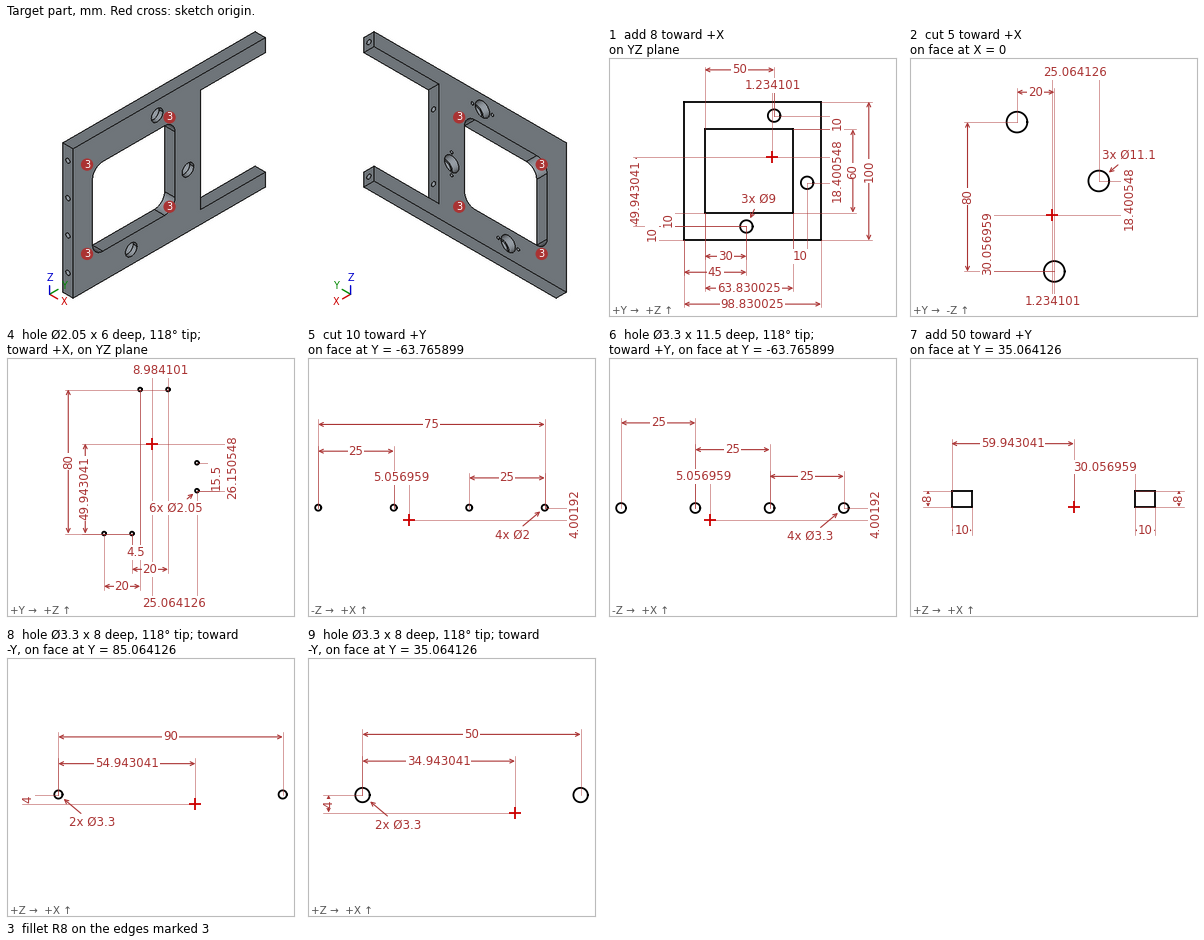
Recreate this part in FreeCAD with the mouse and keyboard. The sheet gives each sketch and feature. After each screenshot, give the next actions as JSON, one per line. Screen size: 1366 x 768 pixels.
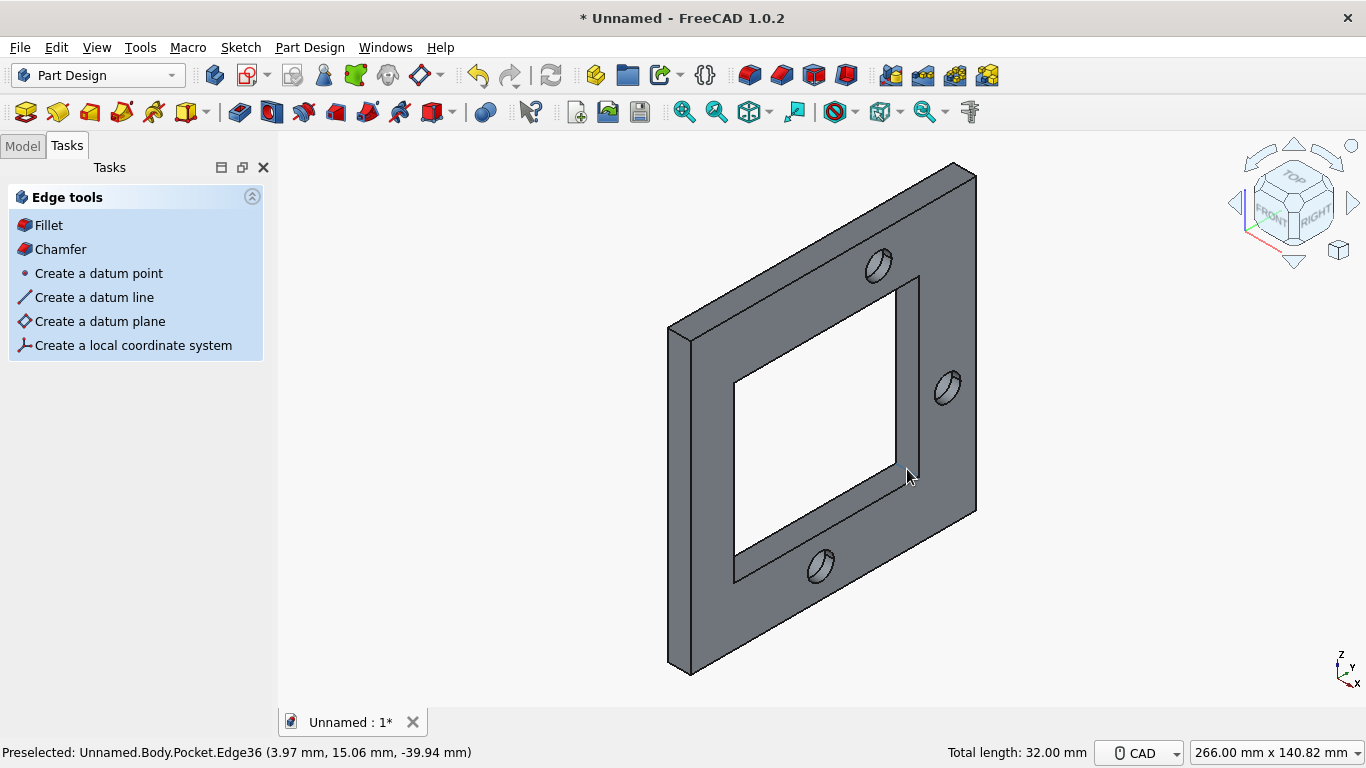
{"action": "left_click", "coordinate": [750, 76]}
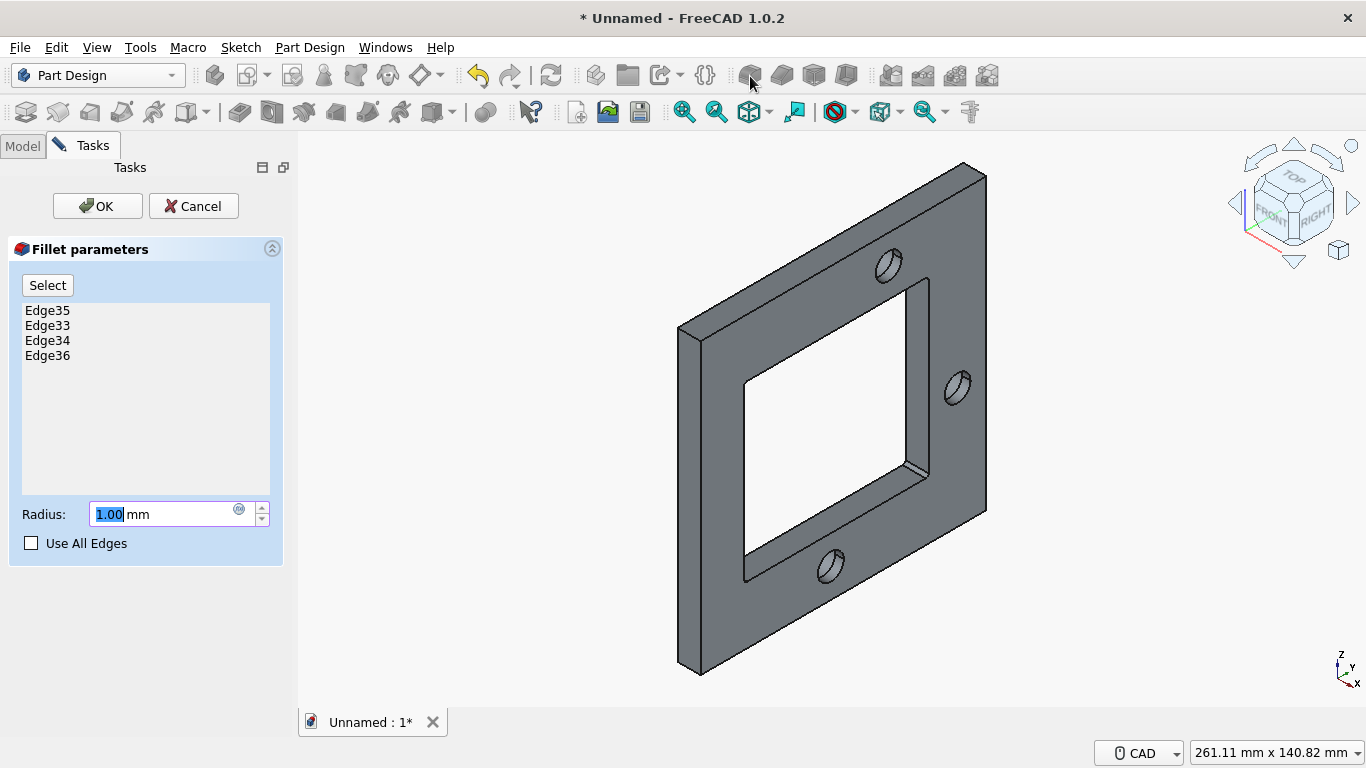
{"action": "type", "text": "8"}
{"action": "key", "text": "Tab"}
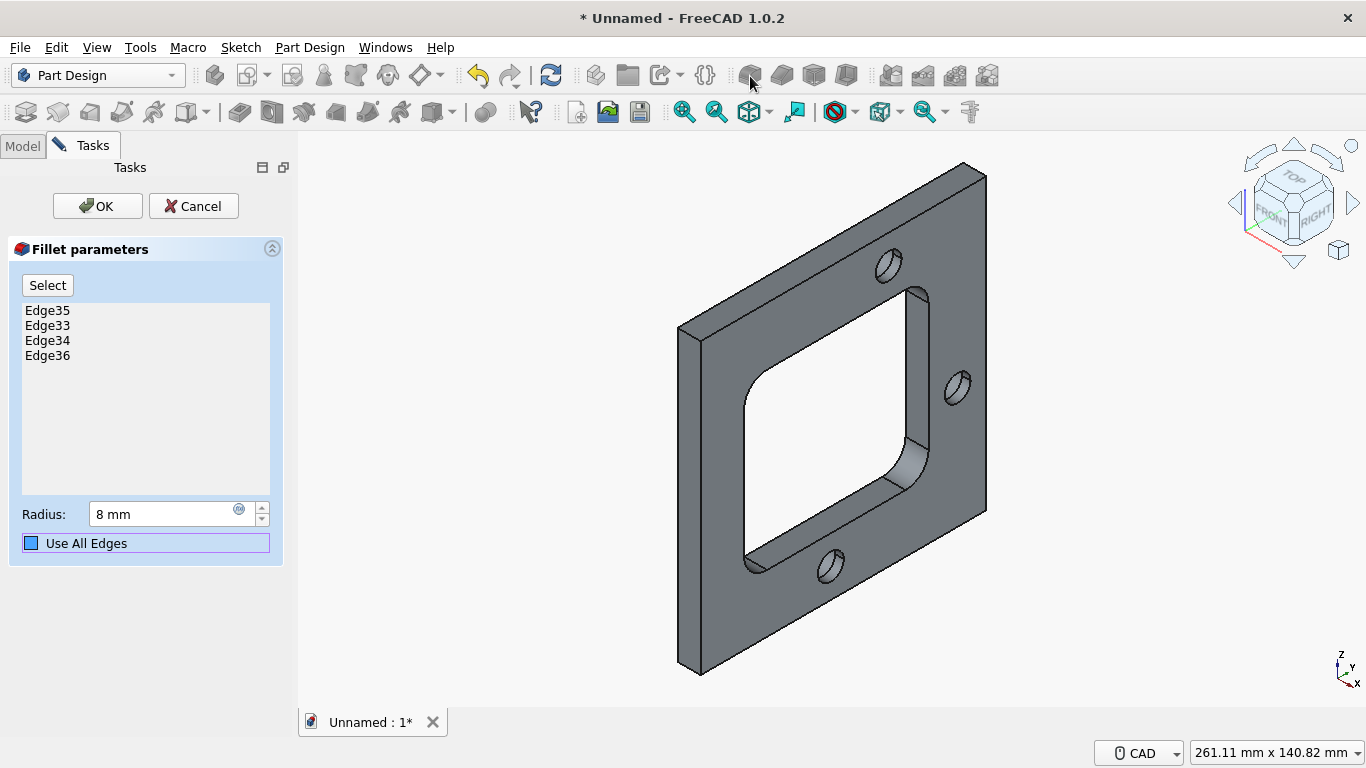
{"action": "left_click", "coordinate": [98, 206]}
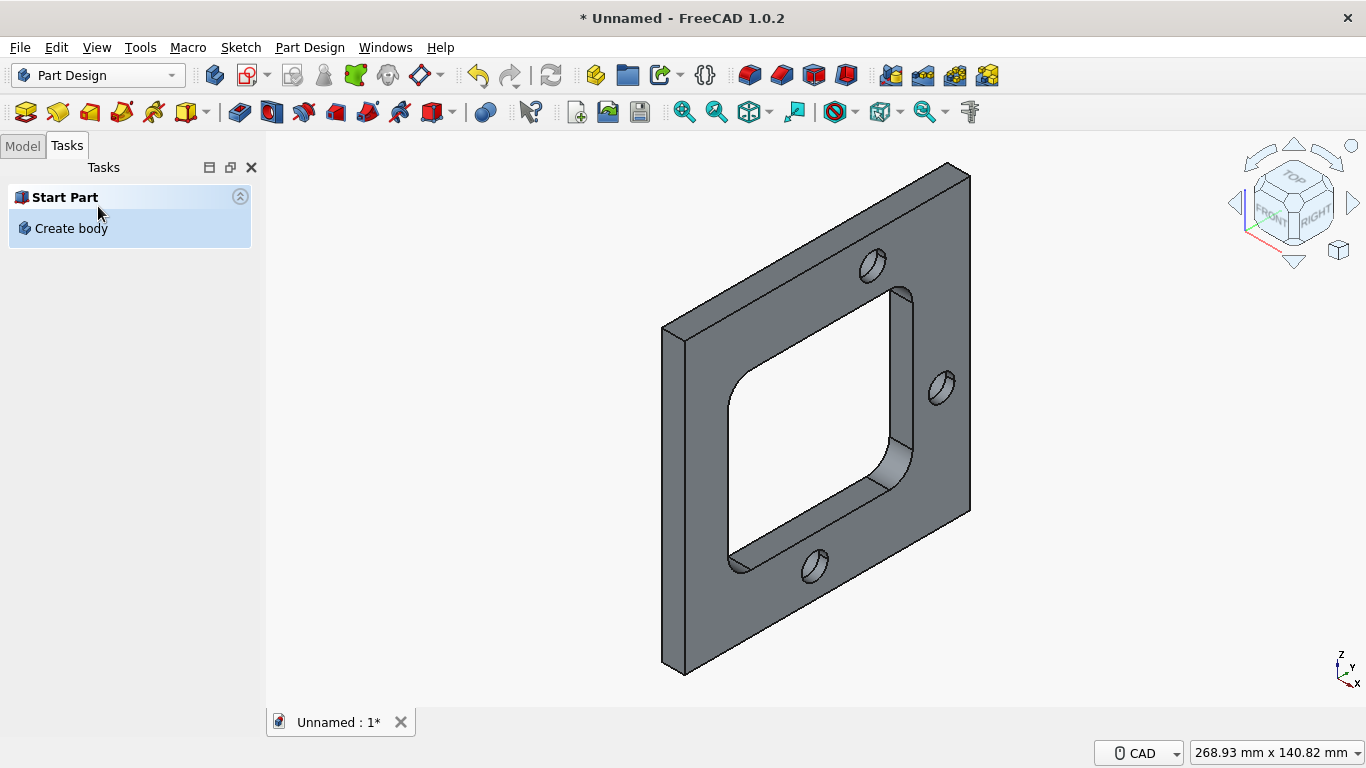
{"action": "left_click", "coordinate": [248, 76]}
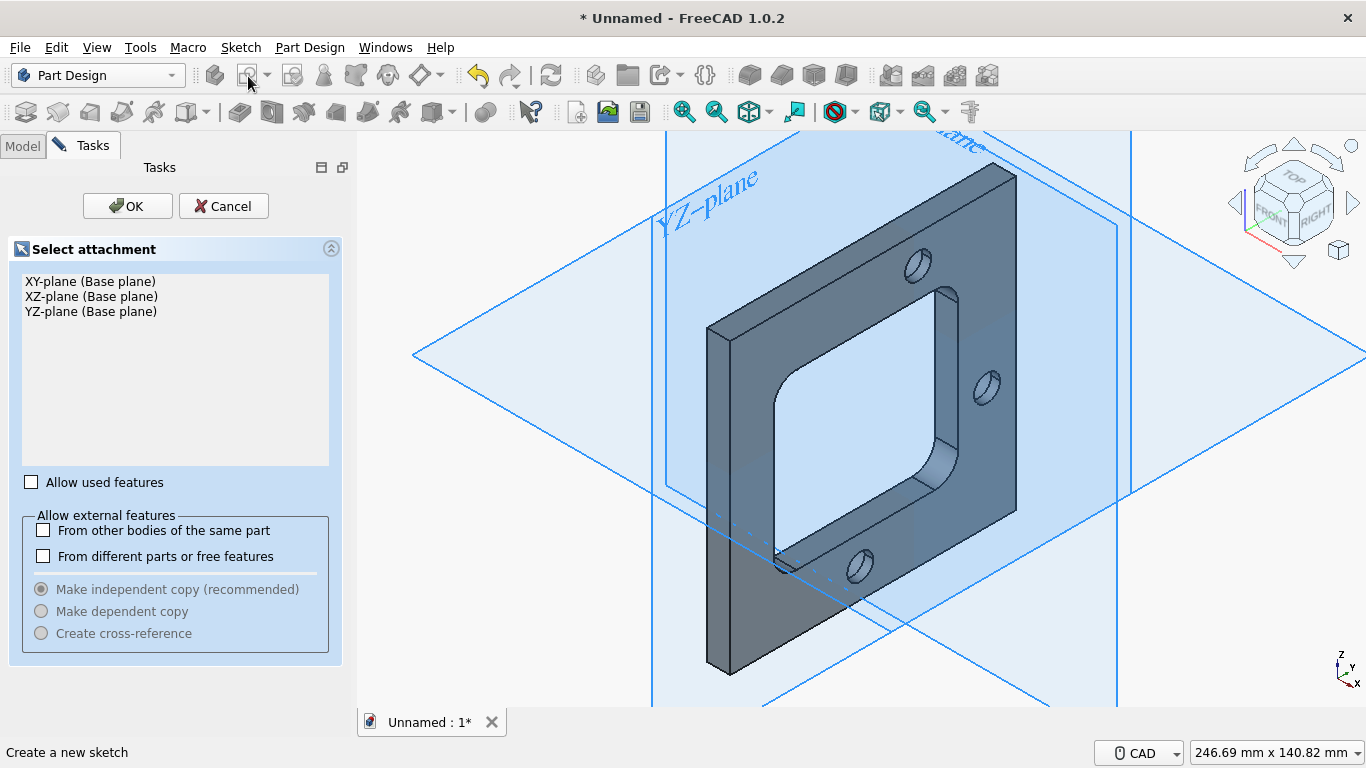
{"action": "left_click", "coordinate": [82, 312]}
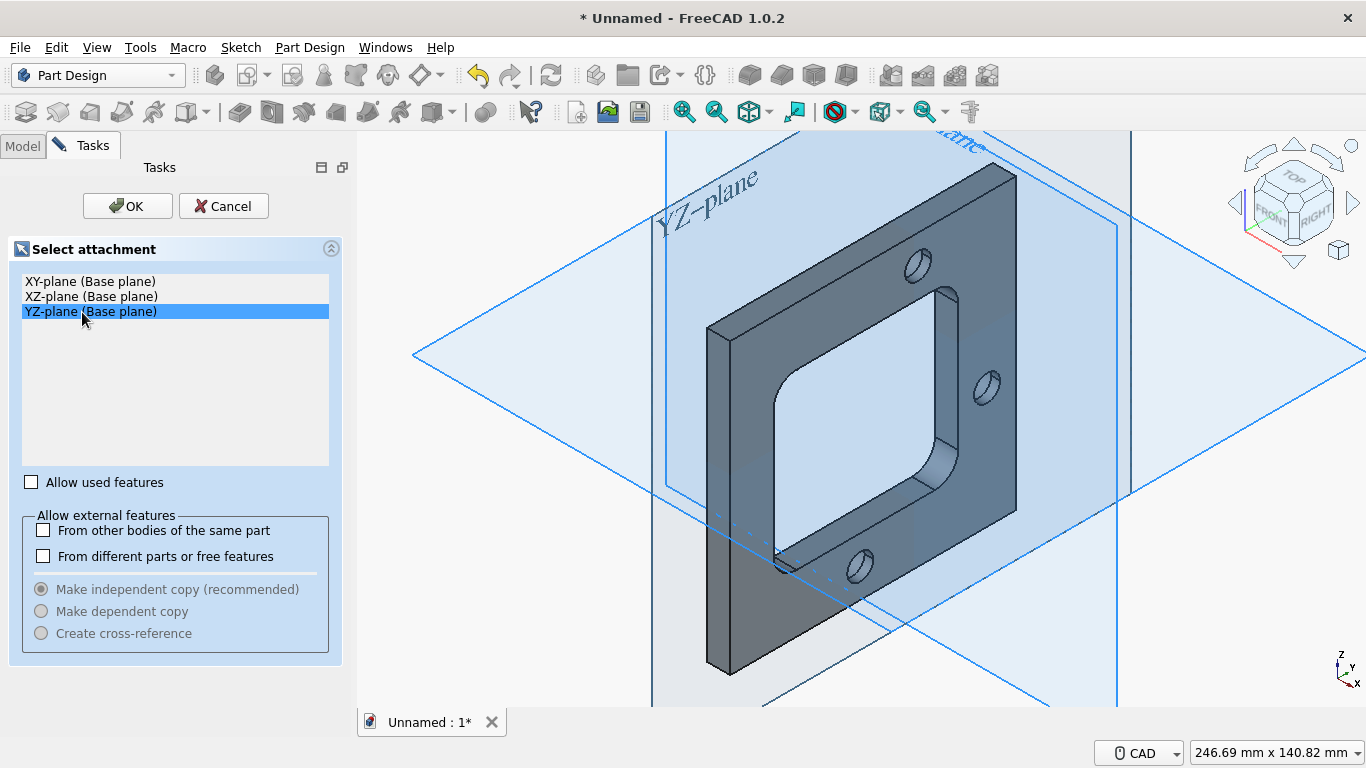
{"action": "left_click", "coordinate": [128, 206]}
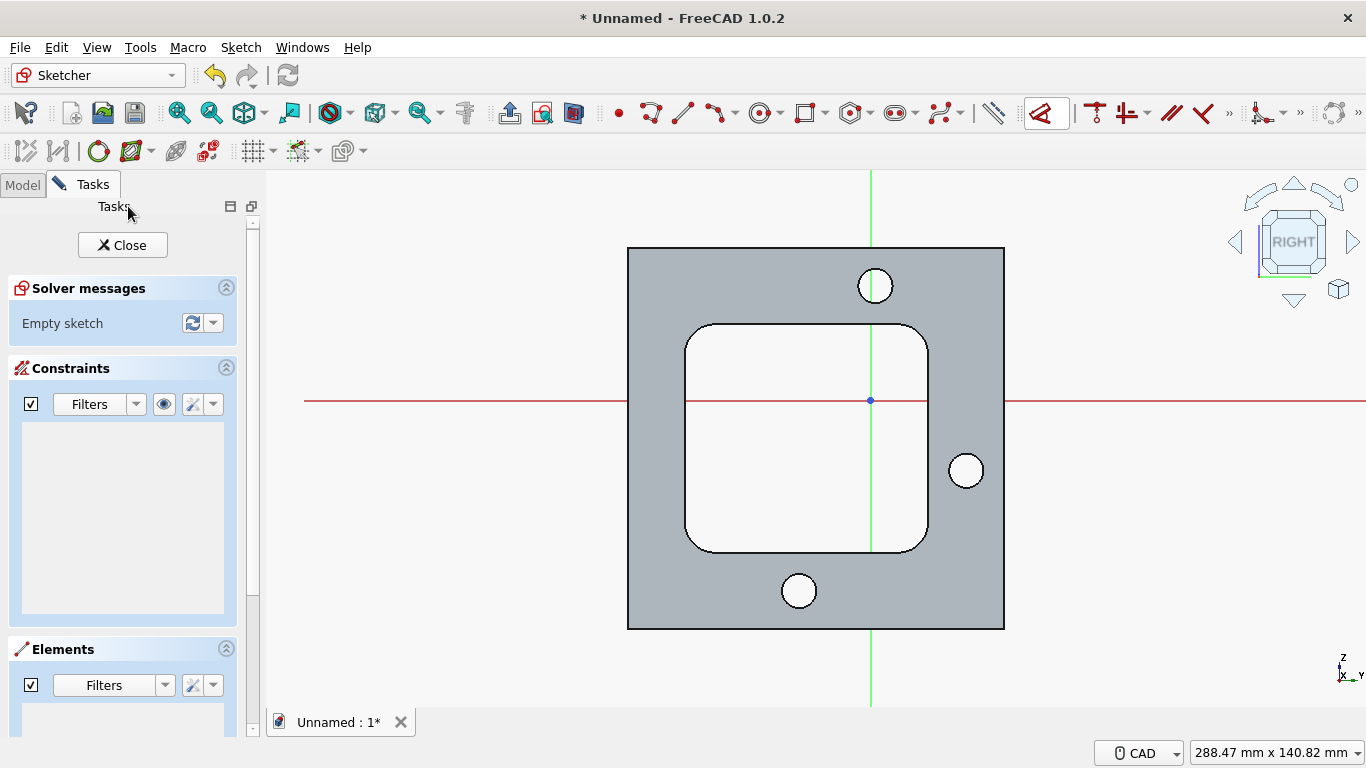
{"action": "left_click", "coordinate": [574, 114]}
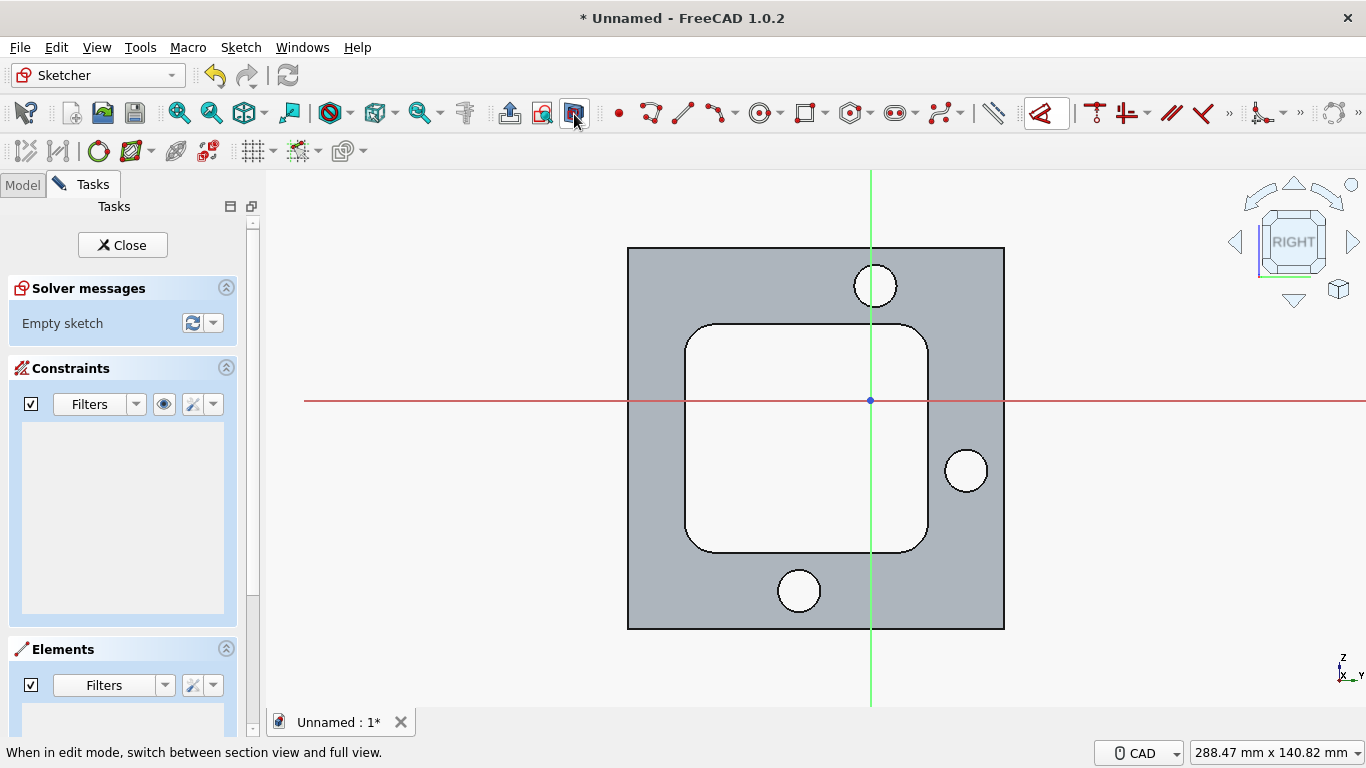
{"action": "left_click", "coordinate": [760, 114]}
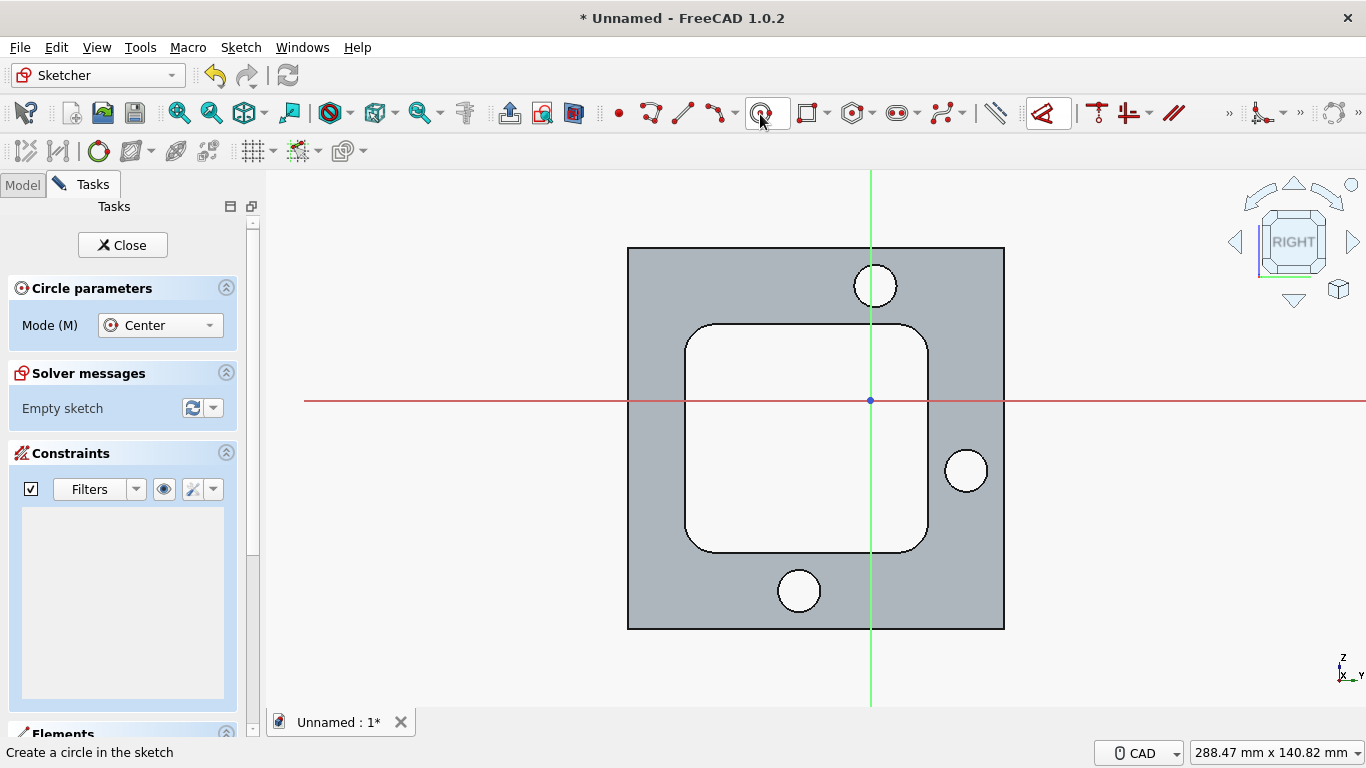
{"action": "scroll", "coordinate": [966, 500], "scroll_direction": "up", "scroll_amount": 9}